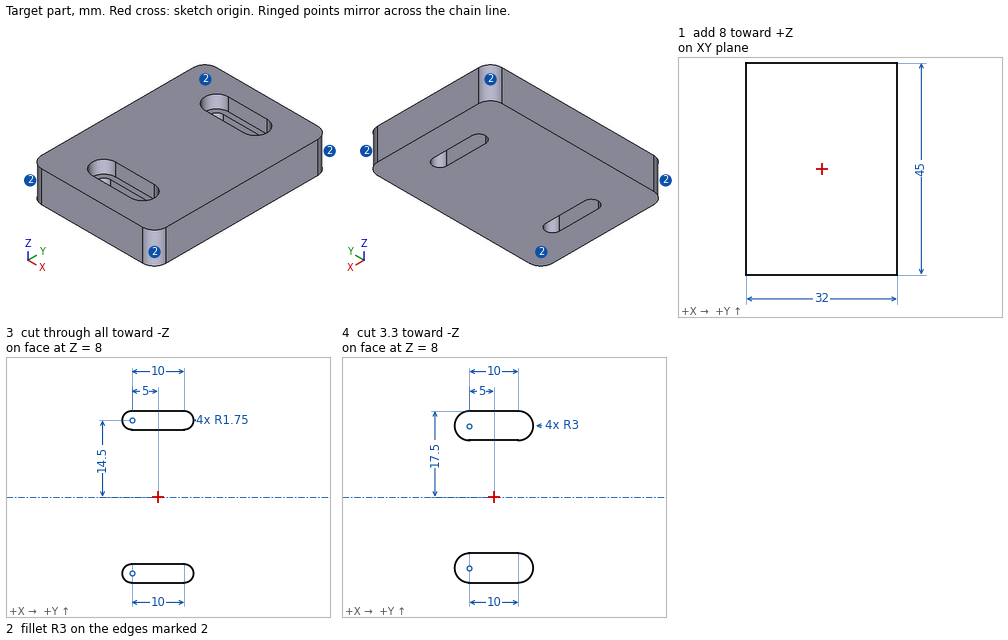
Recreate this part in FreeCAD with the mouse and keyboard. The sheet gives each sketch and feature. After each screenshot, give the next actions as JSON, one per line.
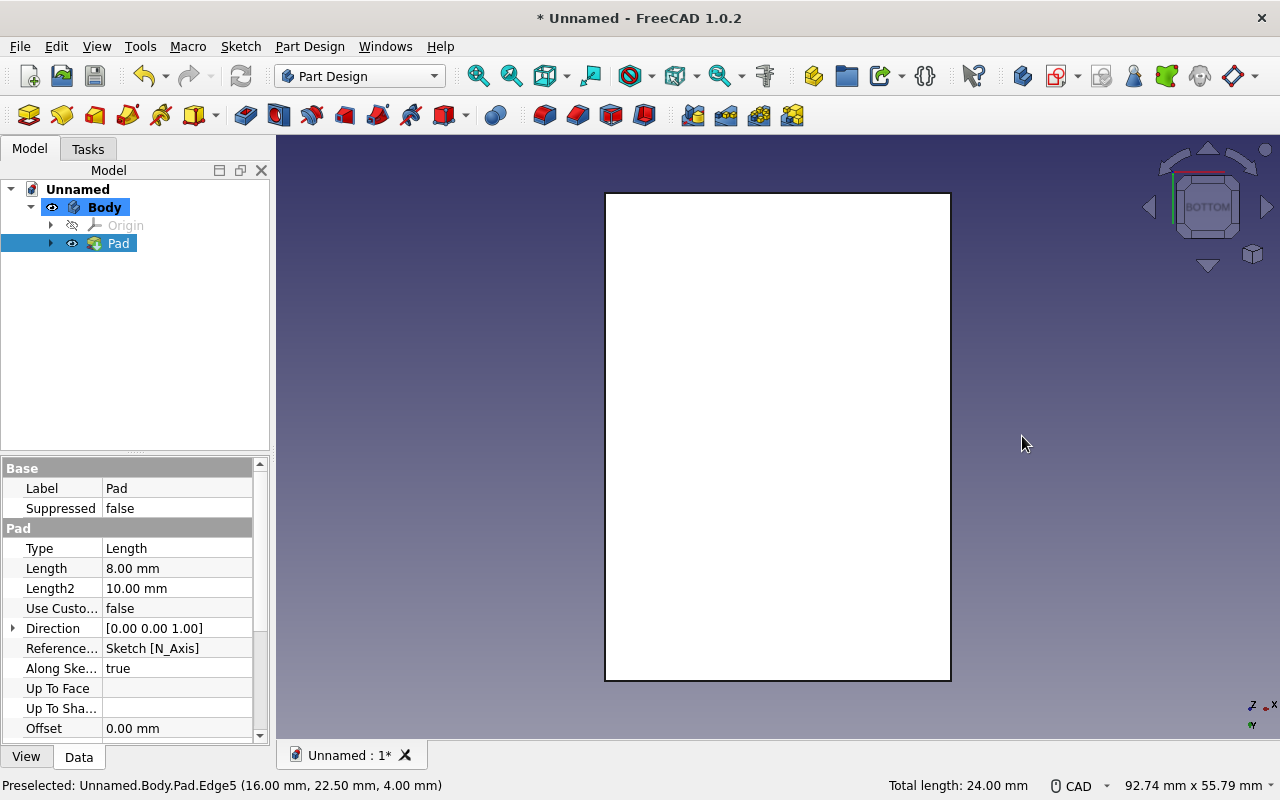
{"action": "key", "text": "4"}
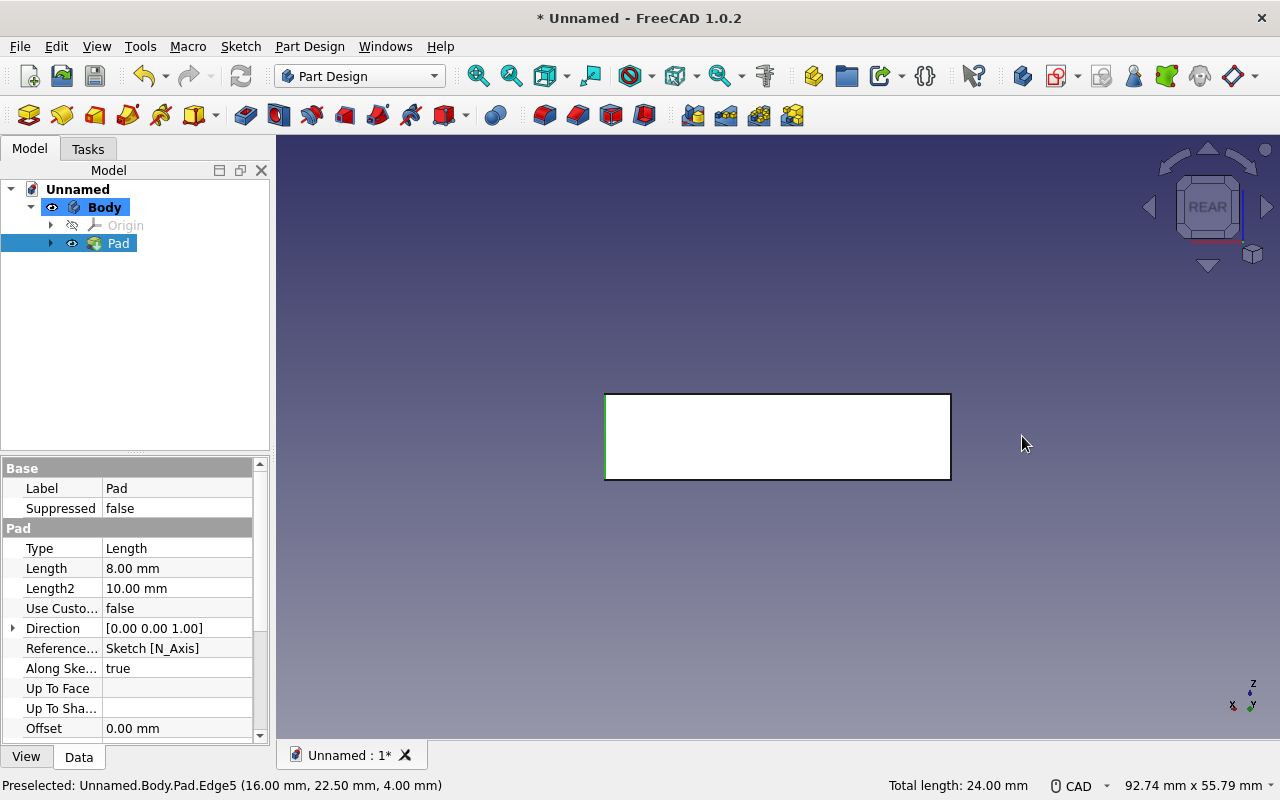
{"action": "left_click", "coordinate": [479, 76]}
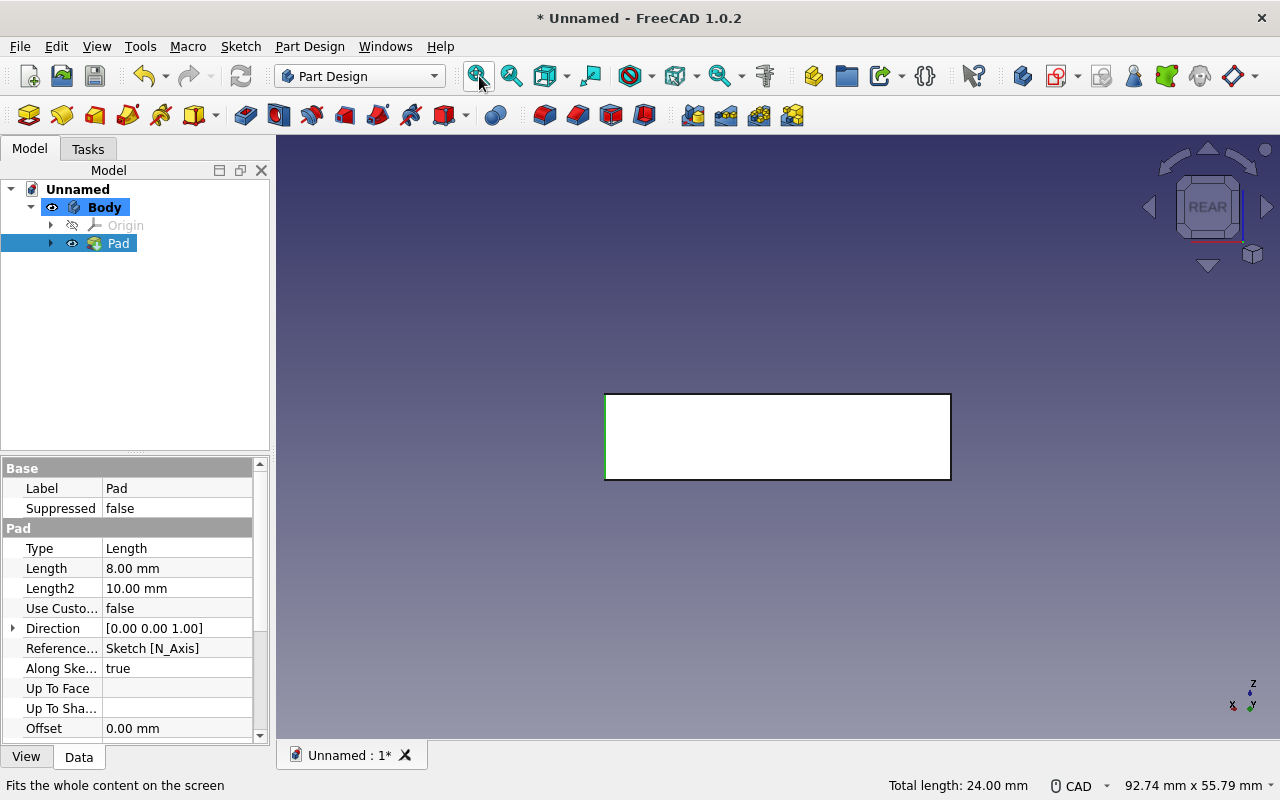
{"action": "left_click", "coordinate": [951, 436], "text": "ctrl"}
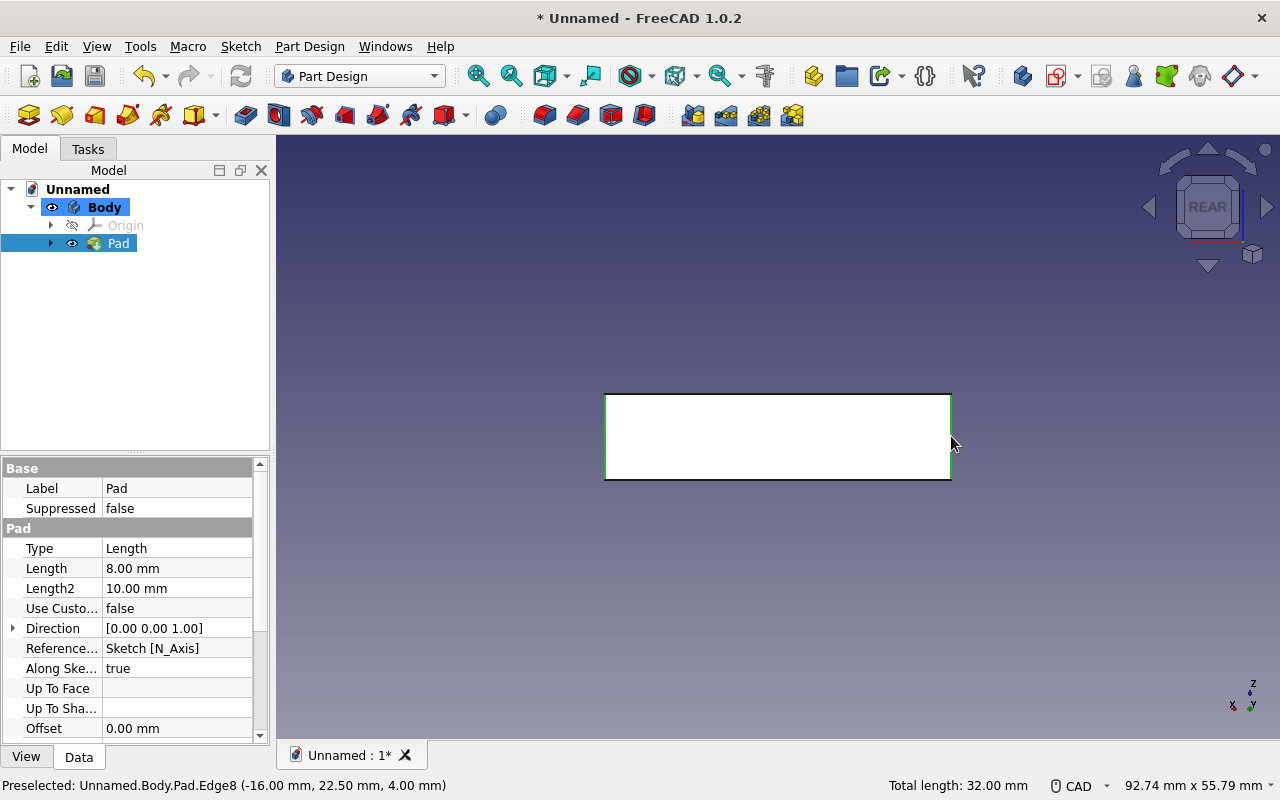
{"action": "left_click", "coordinate": [545, 116]}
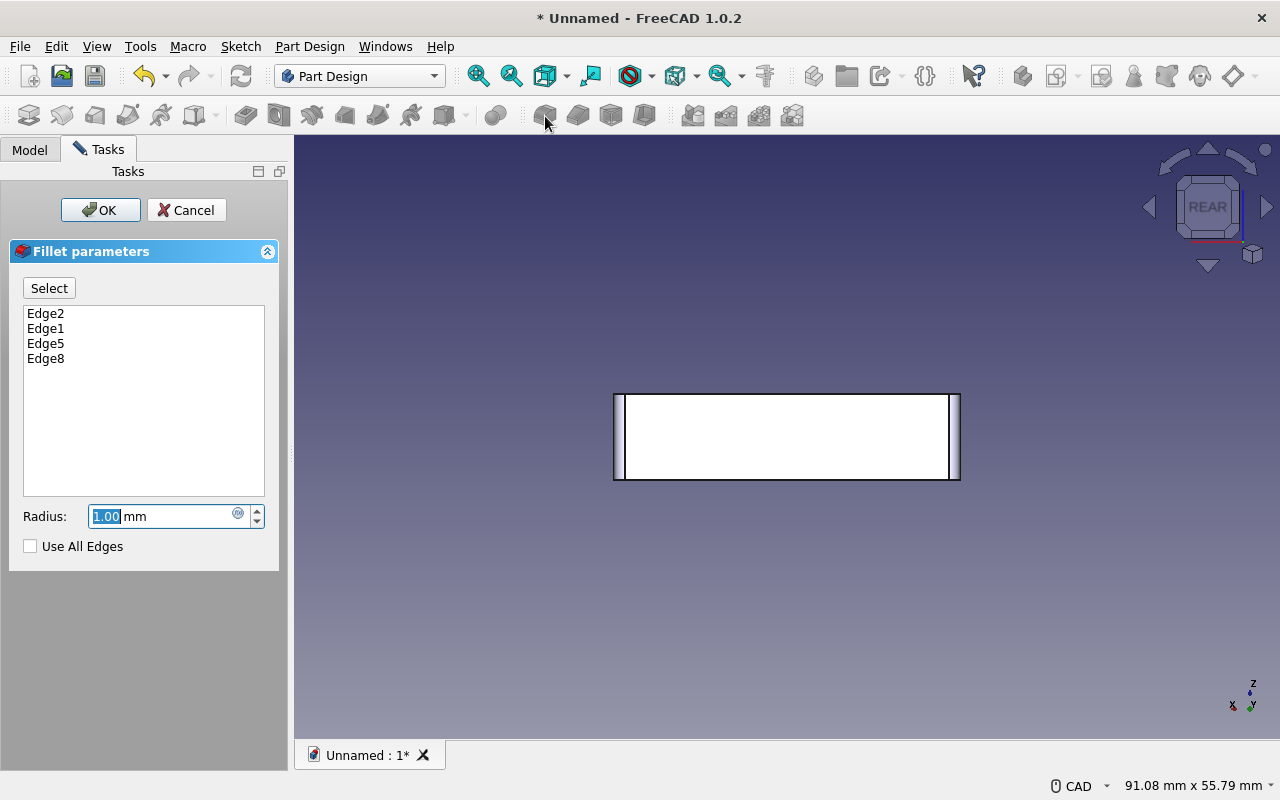
{"action": "type", "text": "3"}
{"action": "key", "text": "Tab"}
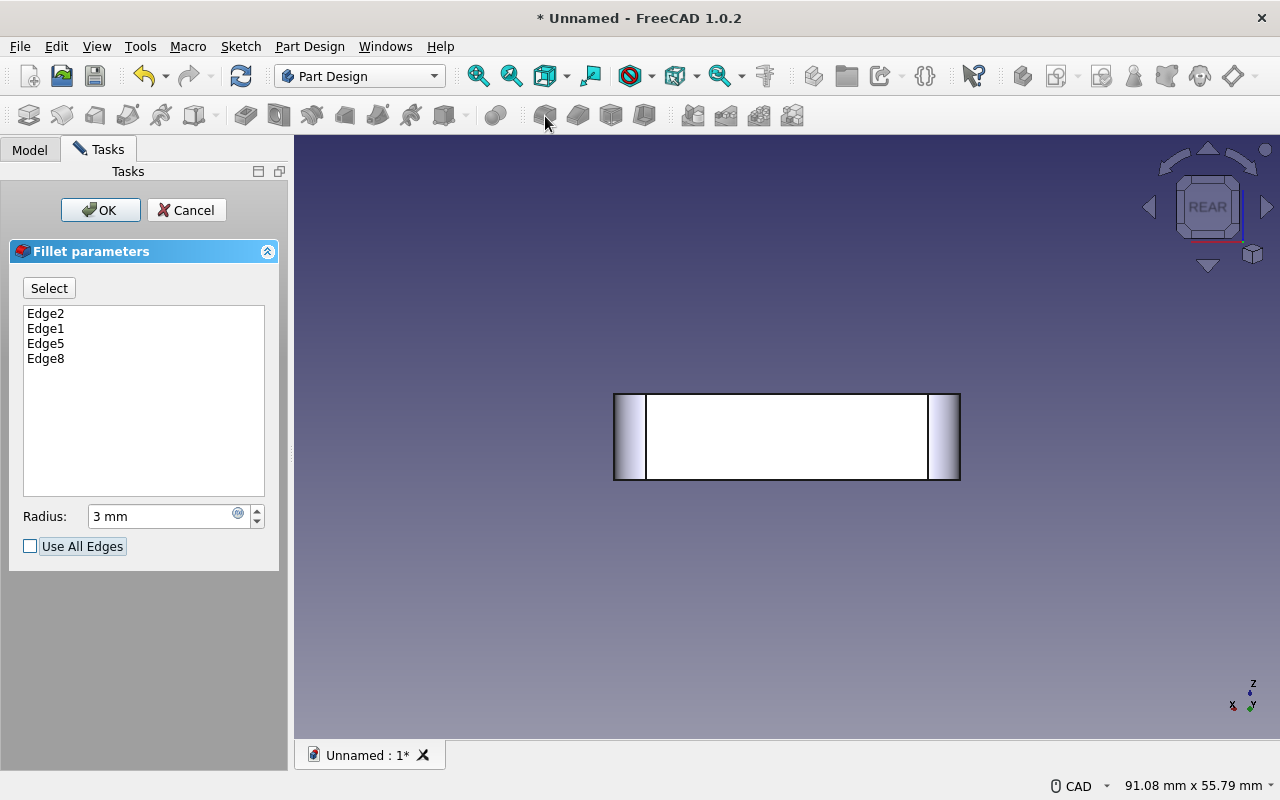
{"action": "left_click", "coordinate": [101, 210]}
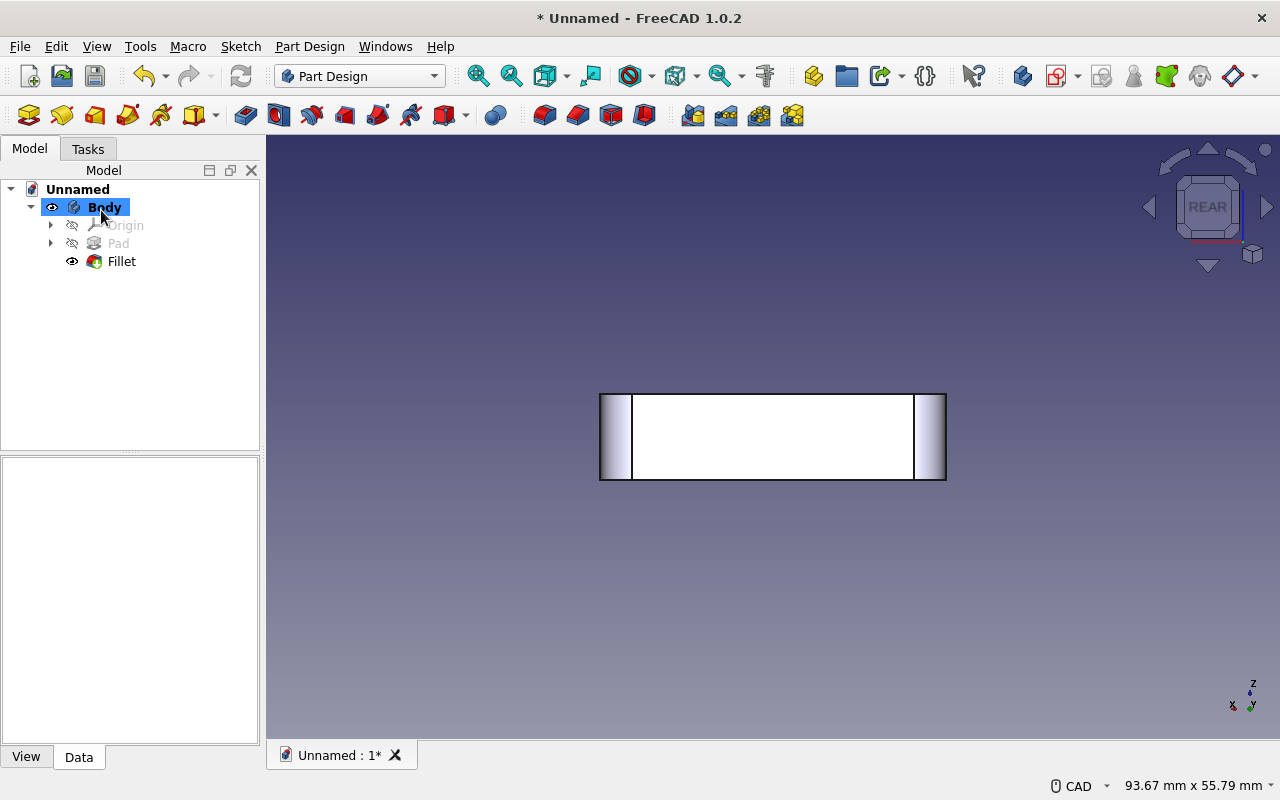
{"action": "left_click", "coordinate": [479, 76]}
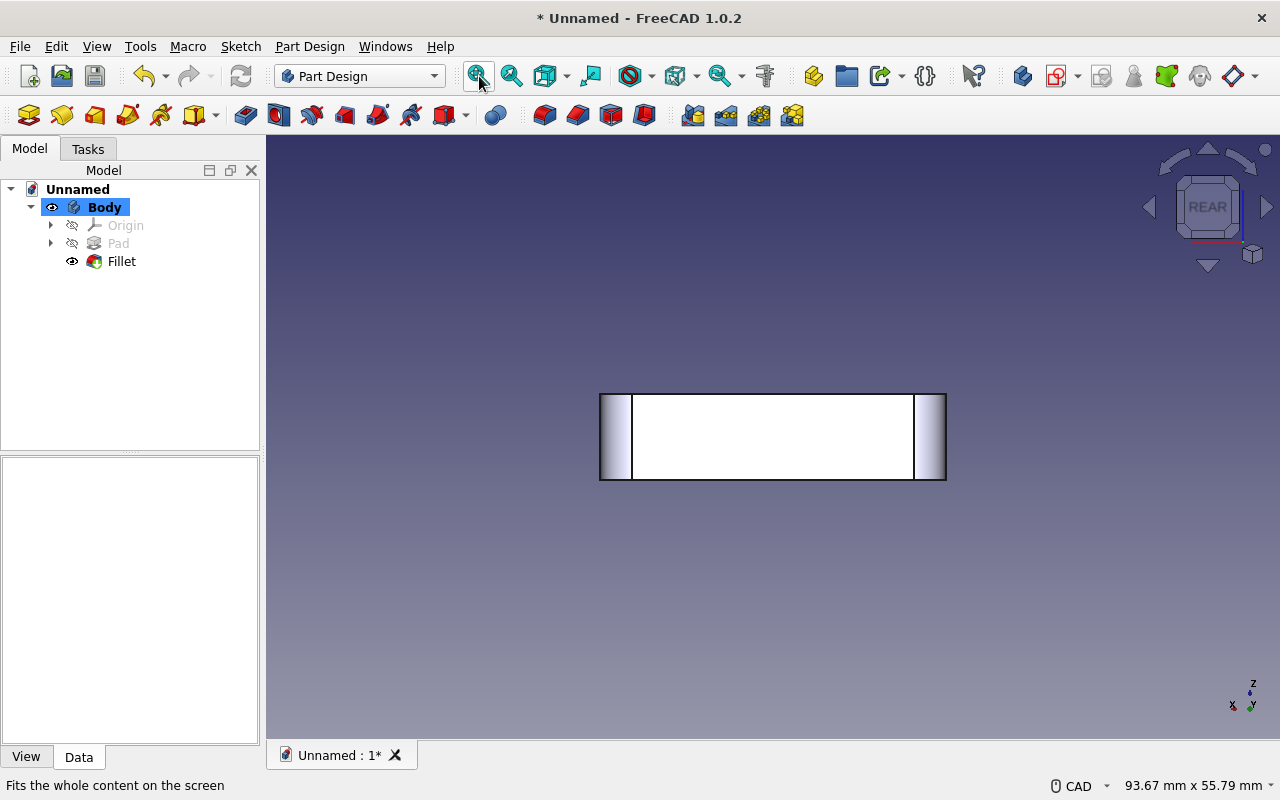
{"action": "key", "text": "0"}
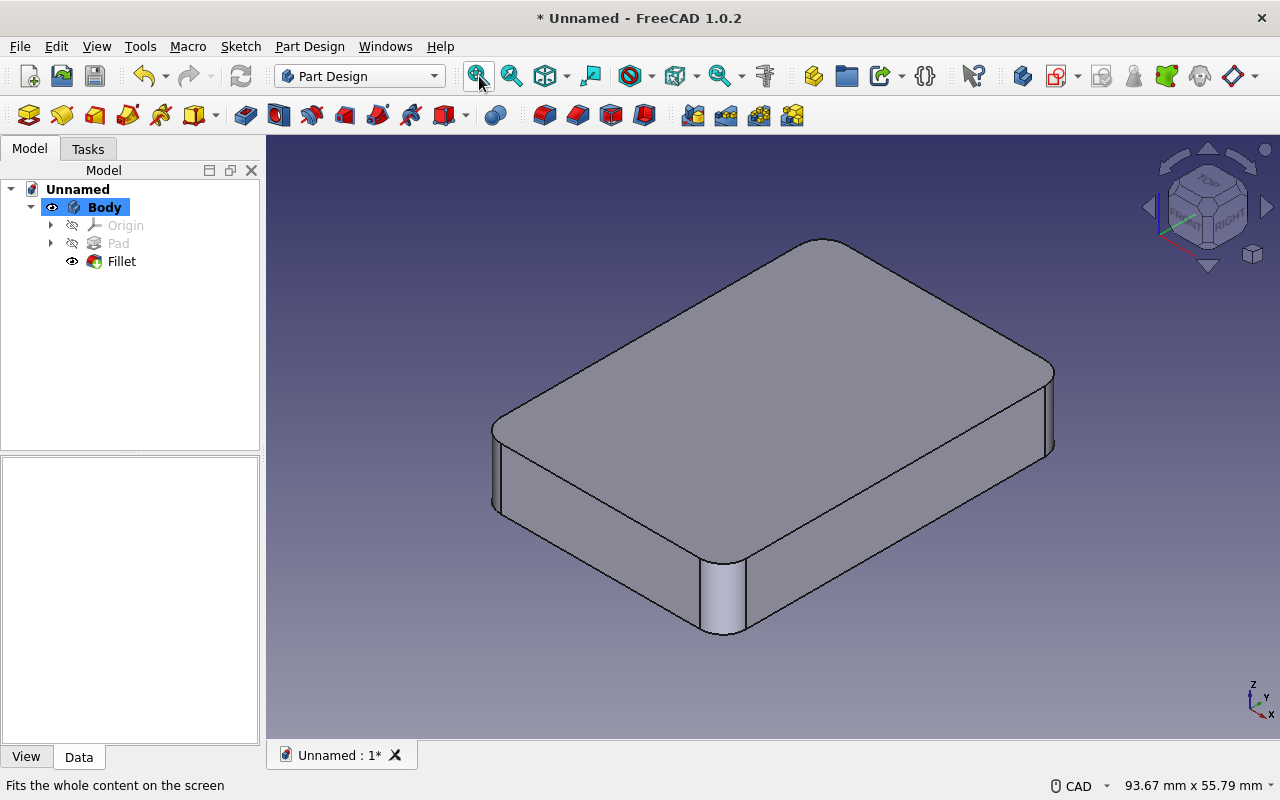
{"action": "left_click", "coordinate": [822, 372]}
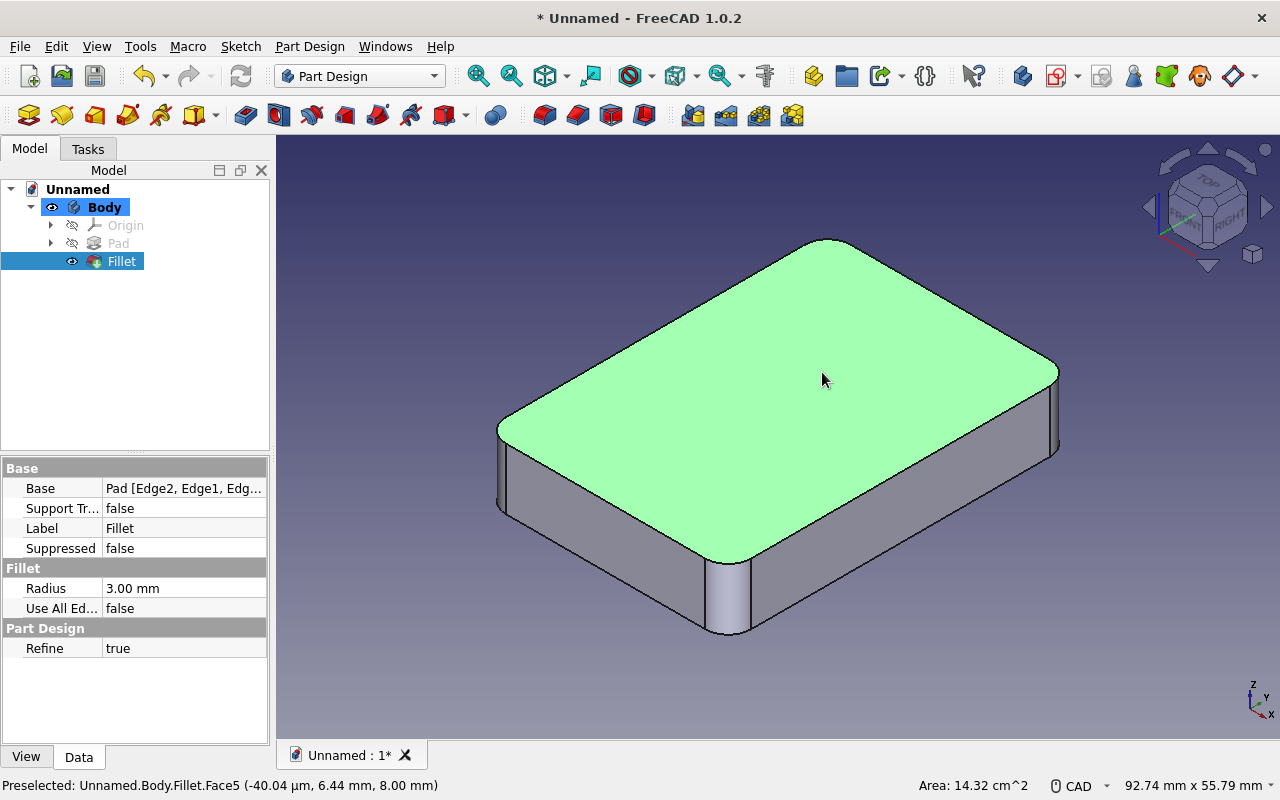
{"action": "left_click", "coordinate": [1056, 76]}